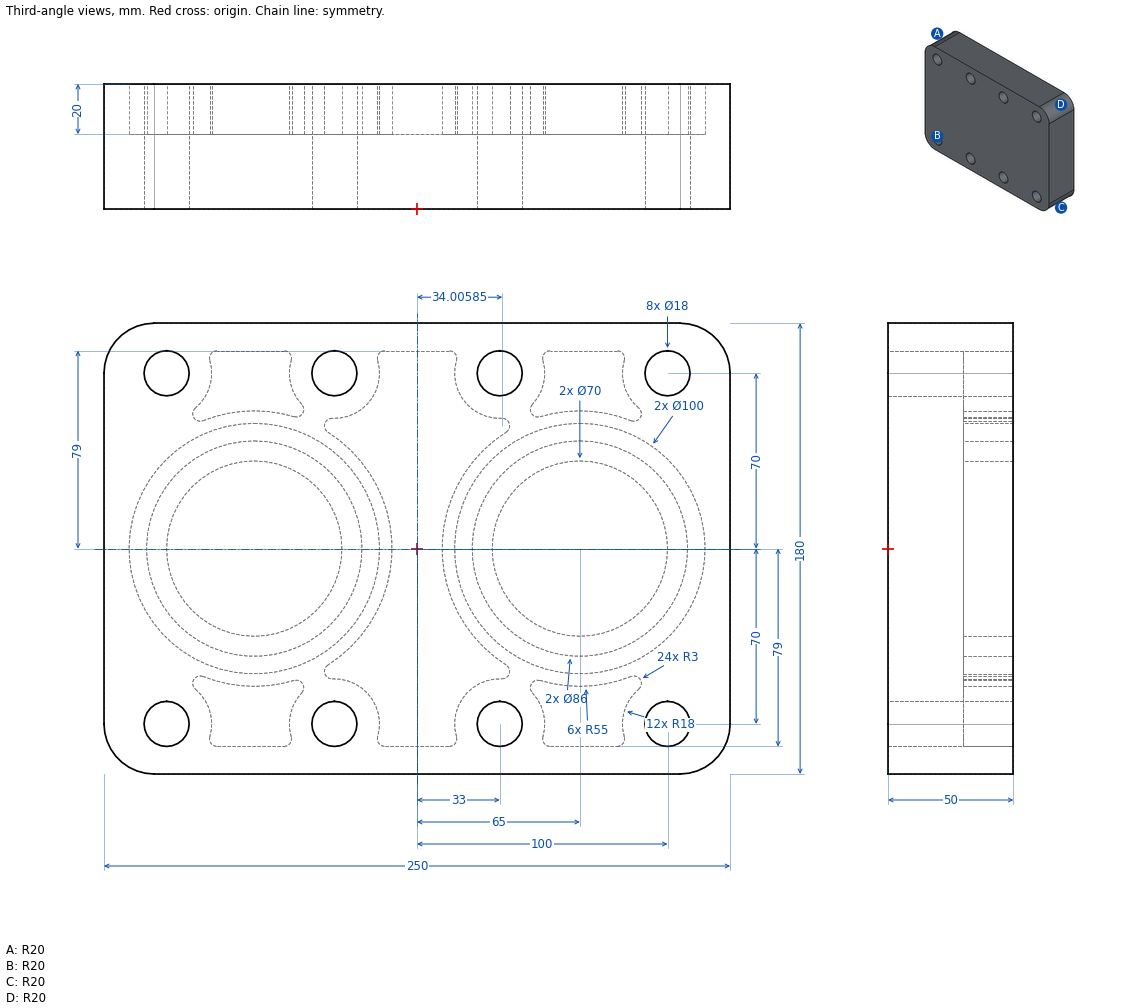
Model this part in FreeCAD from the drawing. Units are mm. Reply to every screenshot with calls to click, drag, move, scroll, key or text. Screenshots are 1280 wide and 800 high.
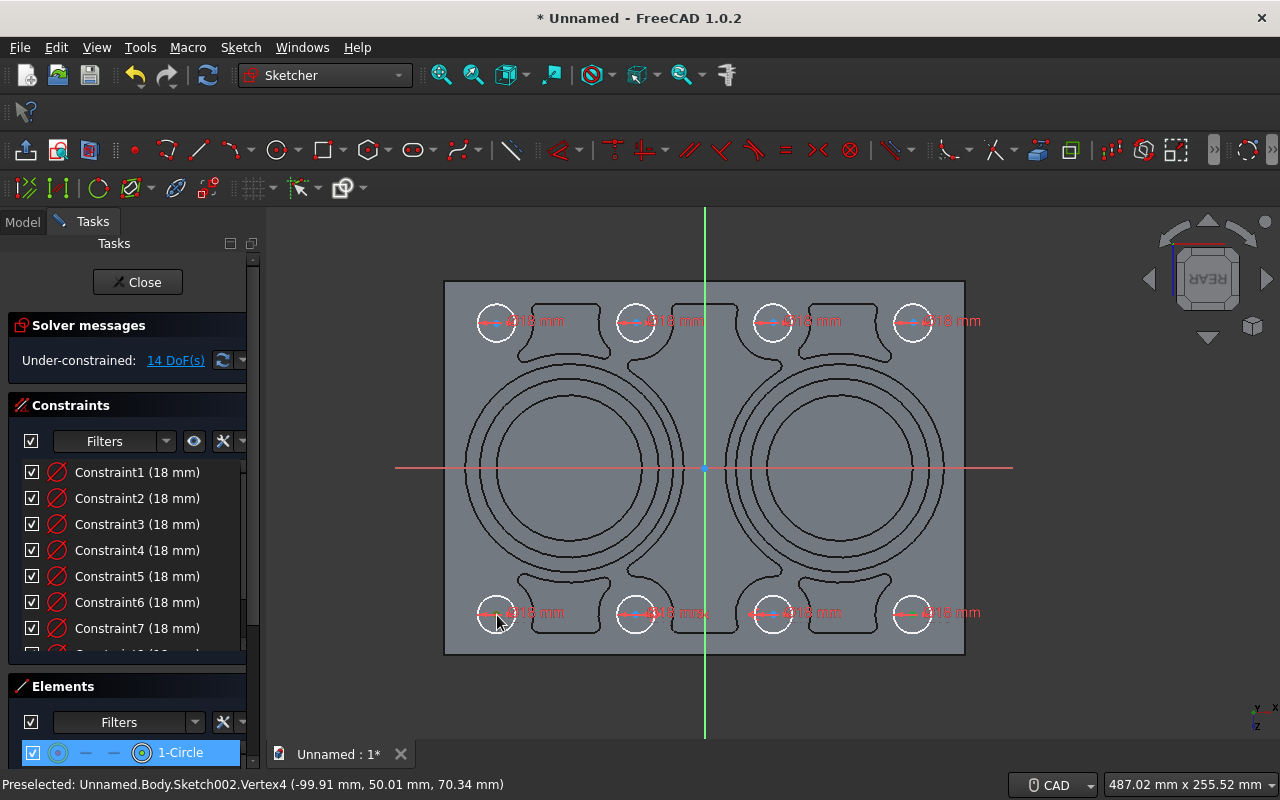
click(705, 677)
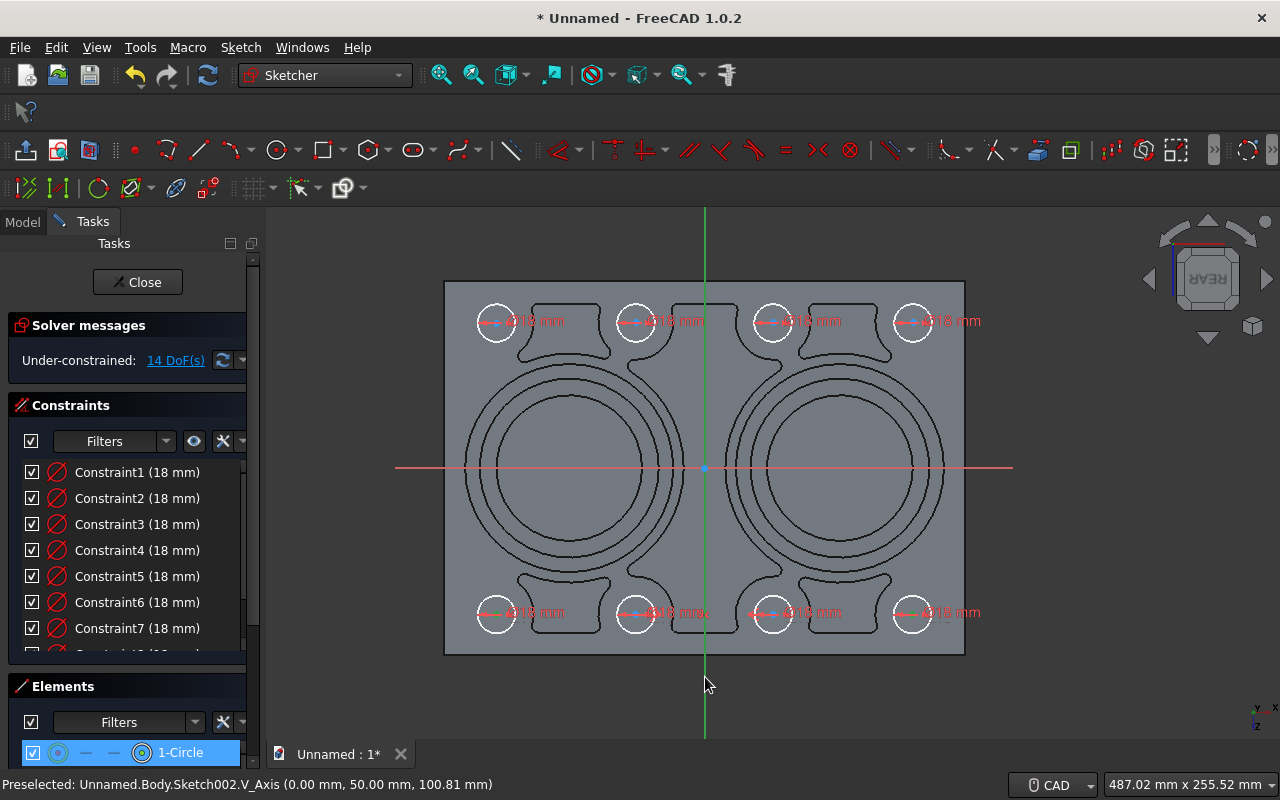
click(818, 150)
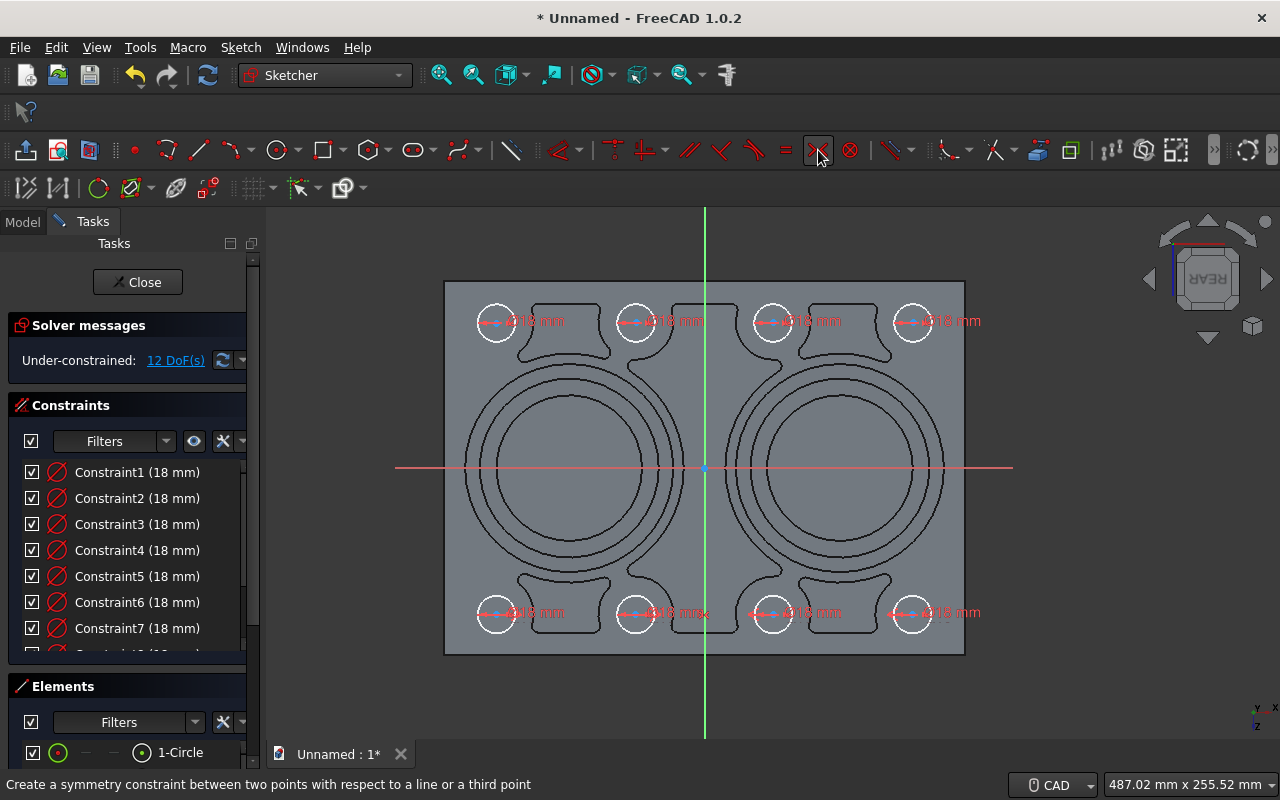
click(497, 615)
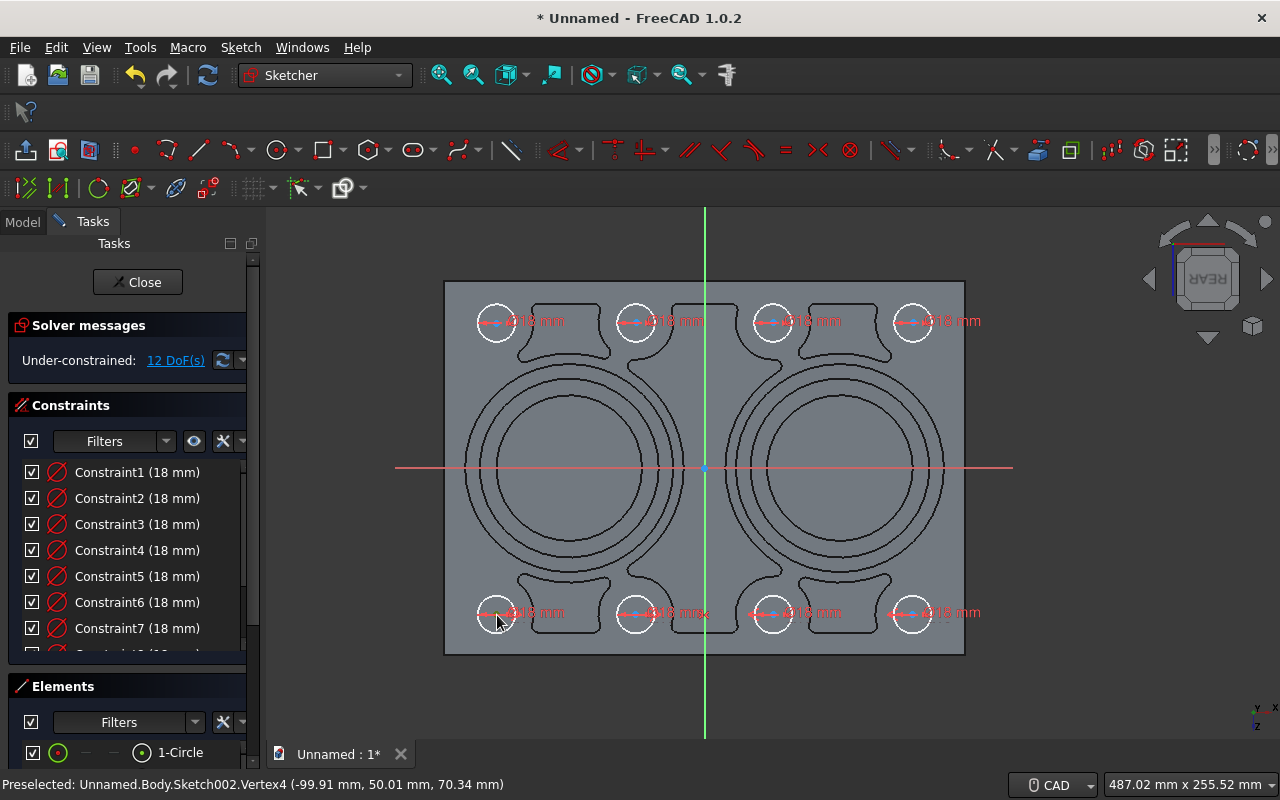
click(497, 323)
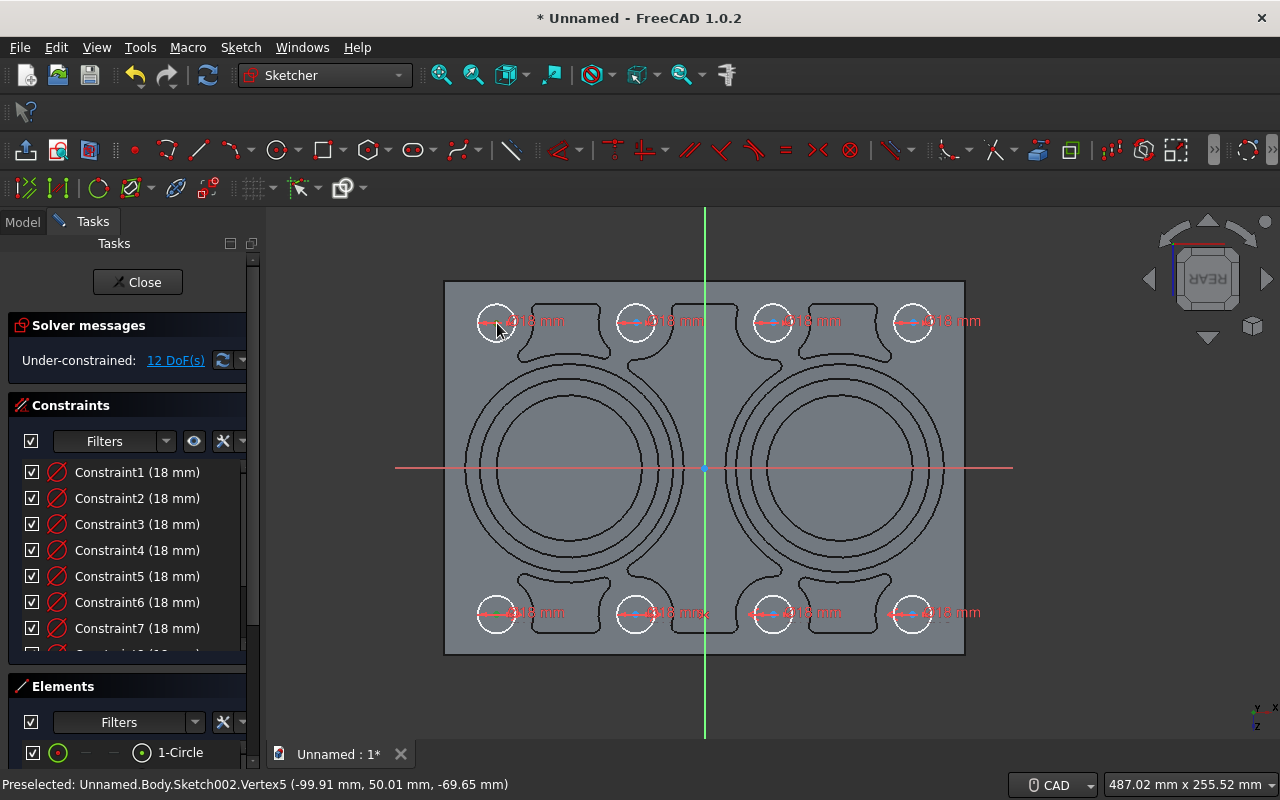
click(411, 468)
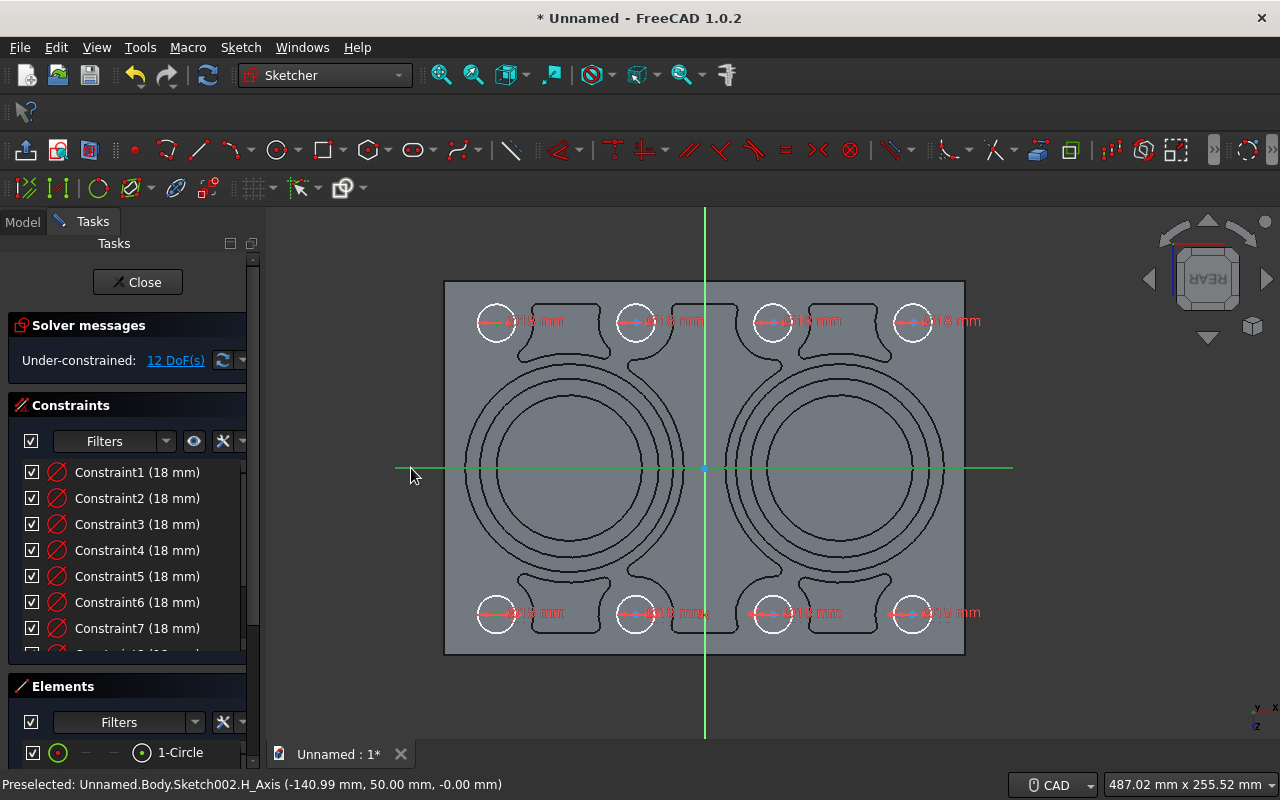
click(818, 150)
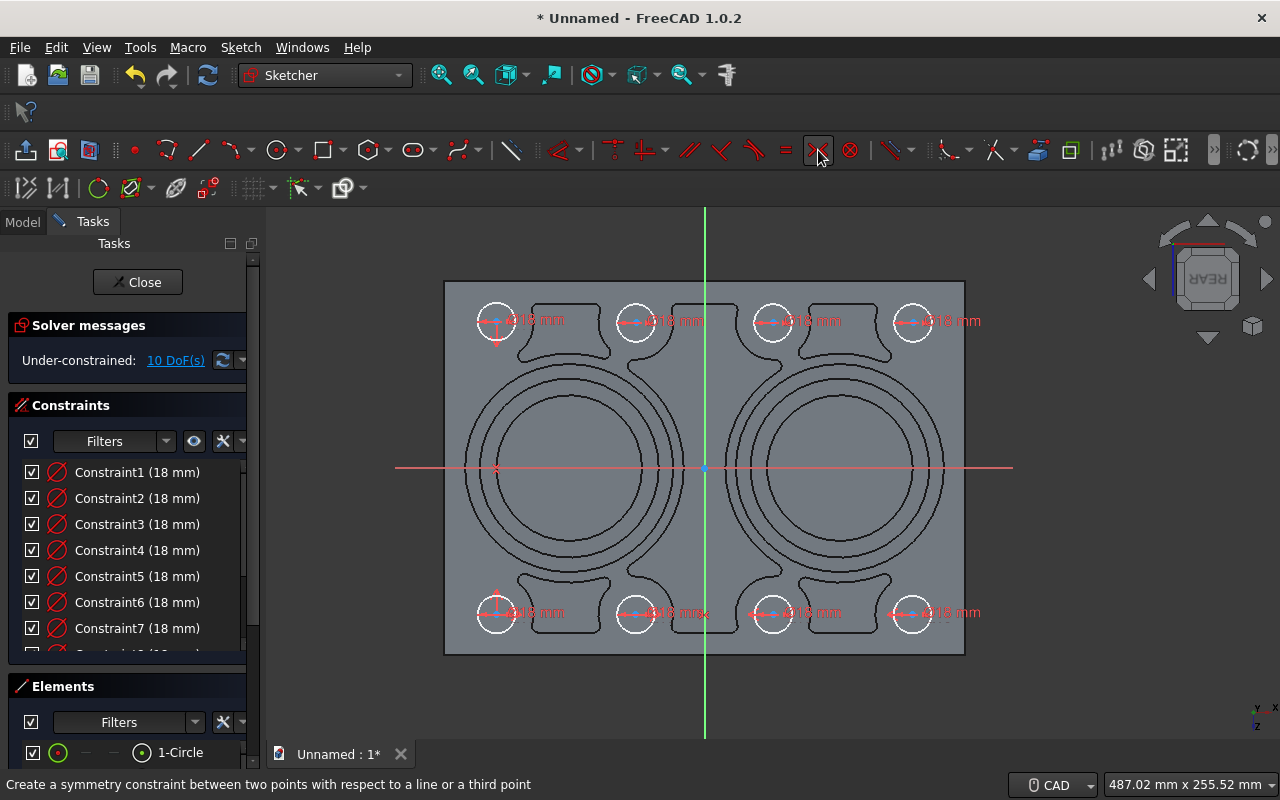
click(636, 615)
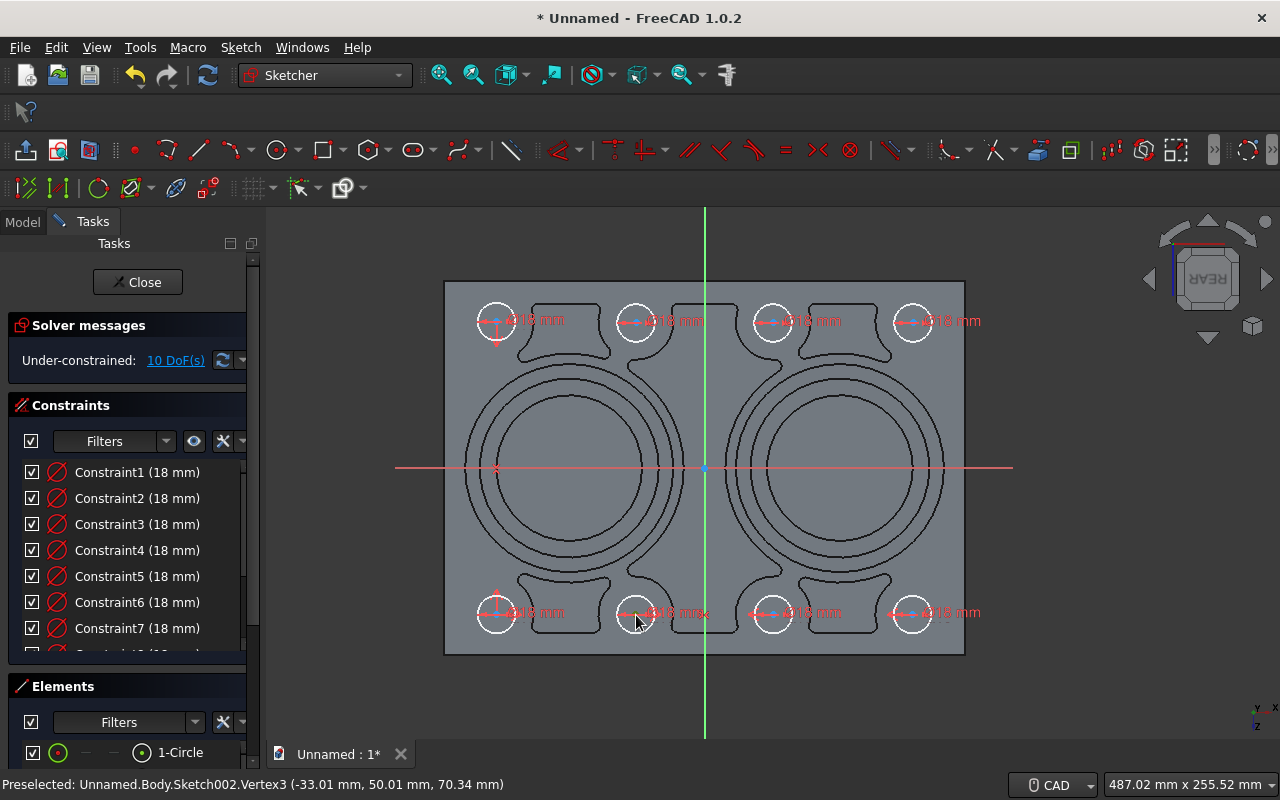
click(636, 323)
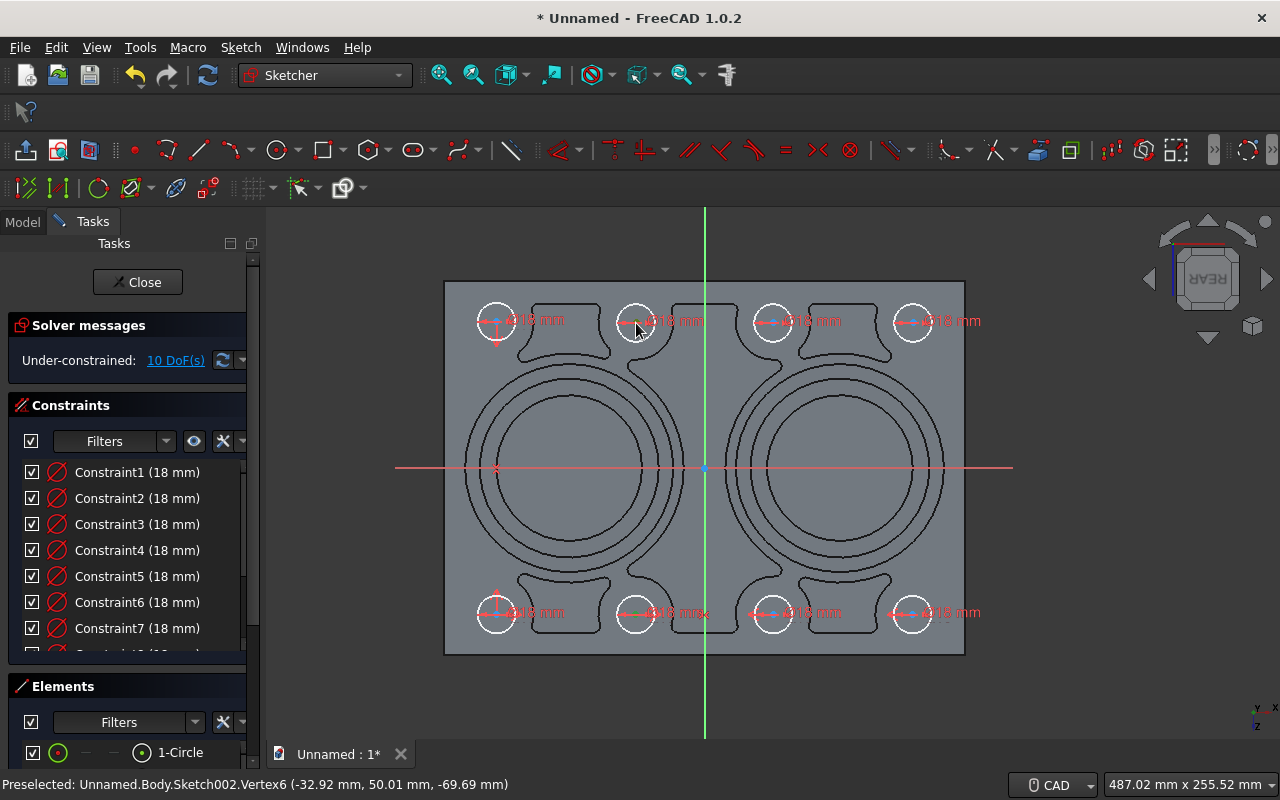
click(411, 468)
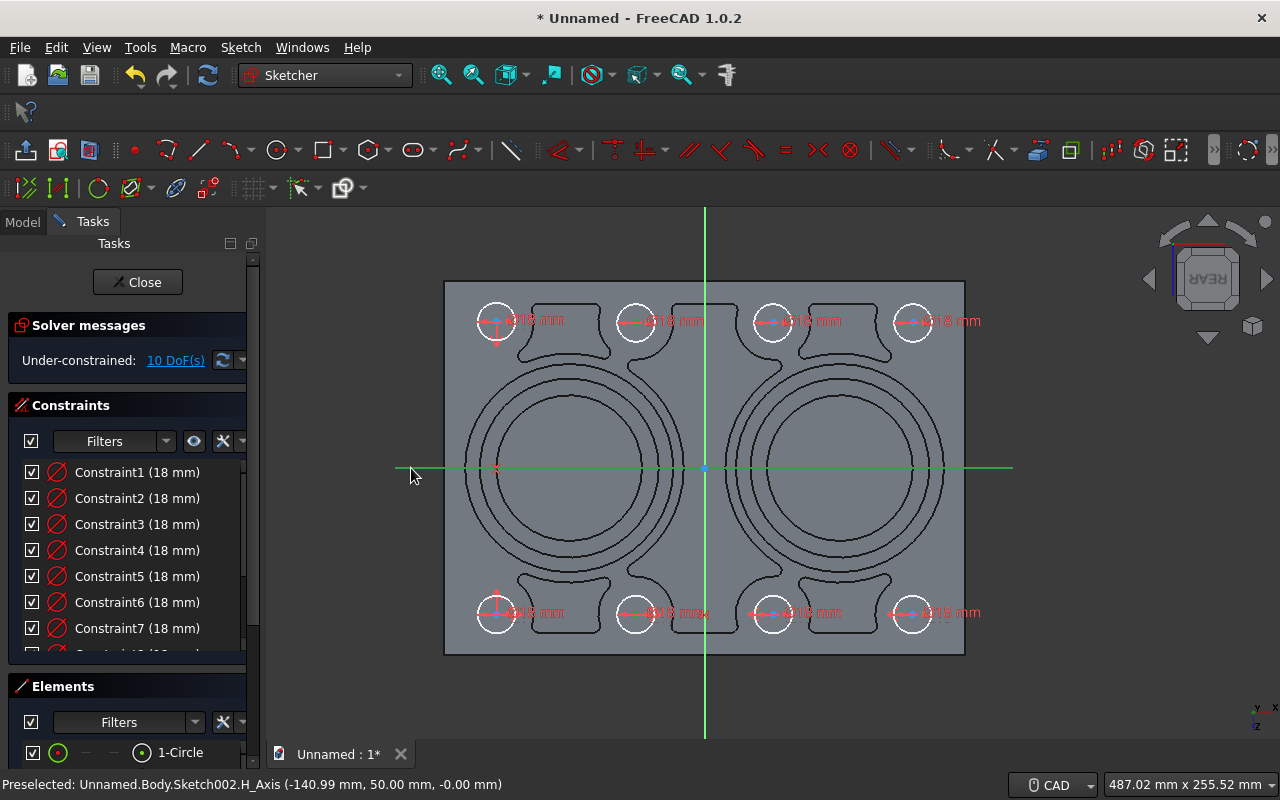
click(818, 150)